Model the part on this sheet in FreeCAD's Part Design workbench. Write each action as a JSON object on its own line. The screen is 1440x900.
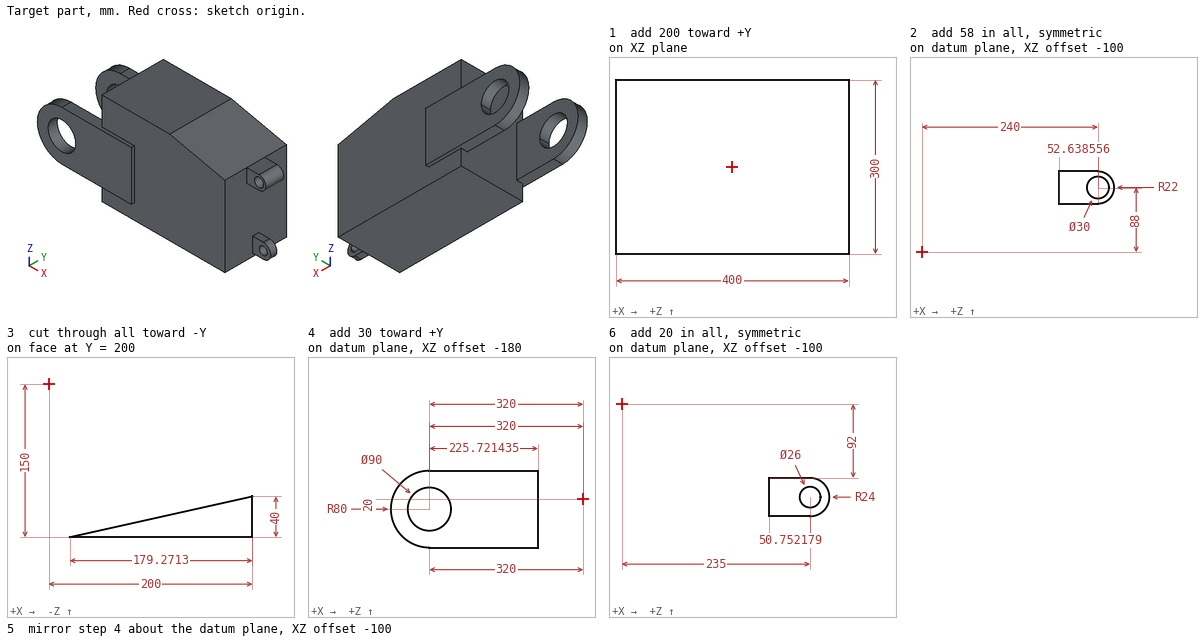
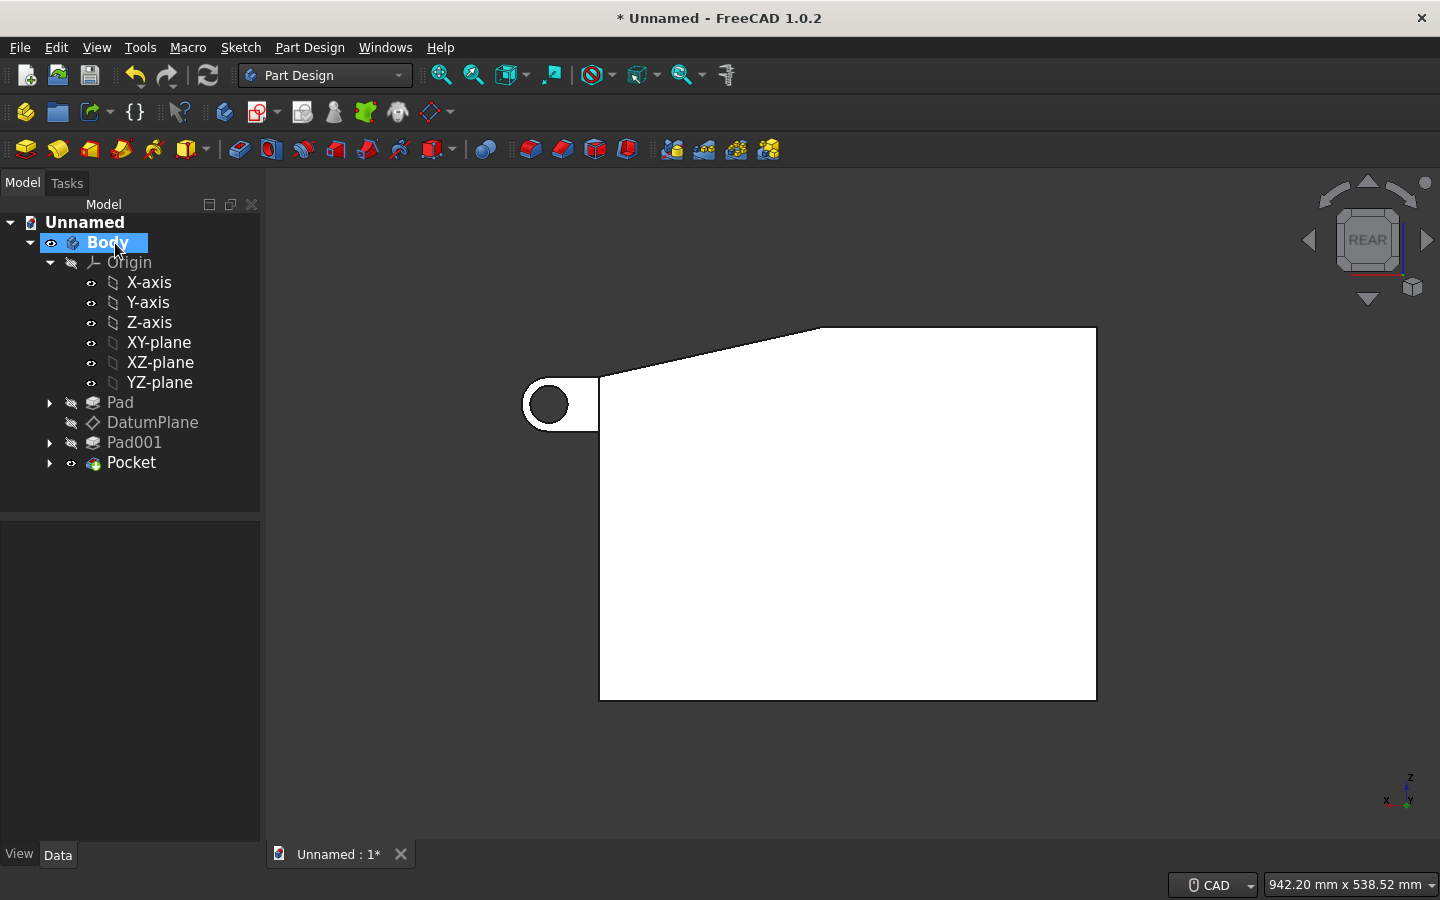
{"action": "left_click", "coordinate": [136, 363]}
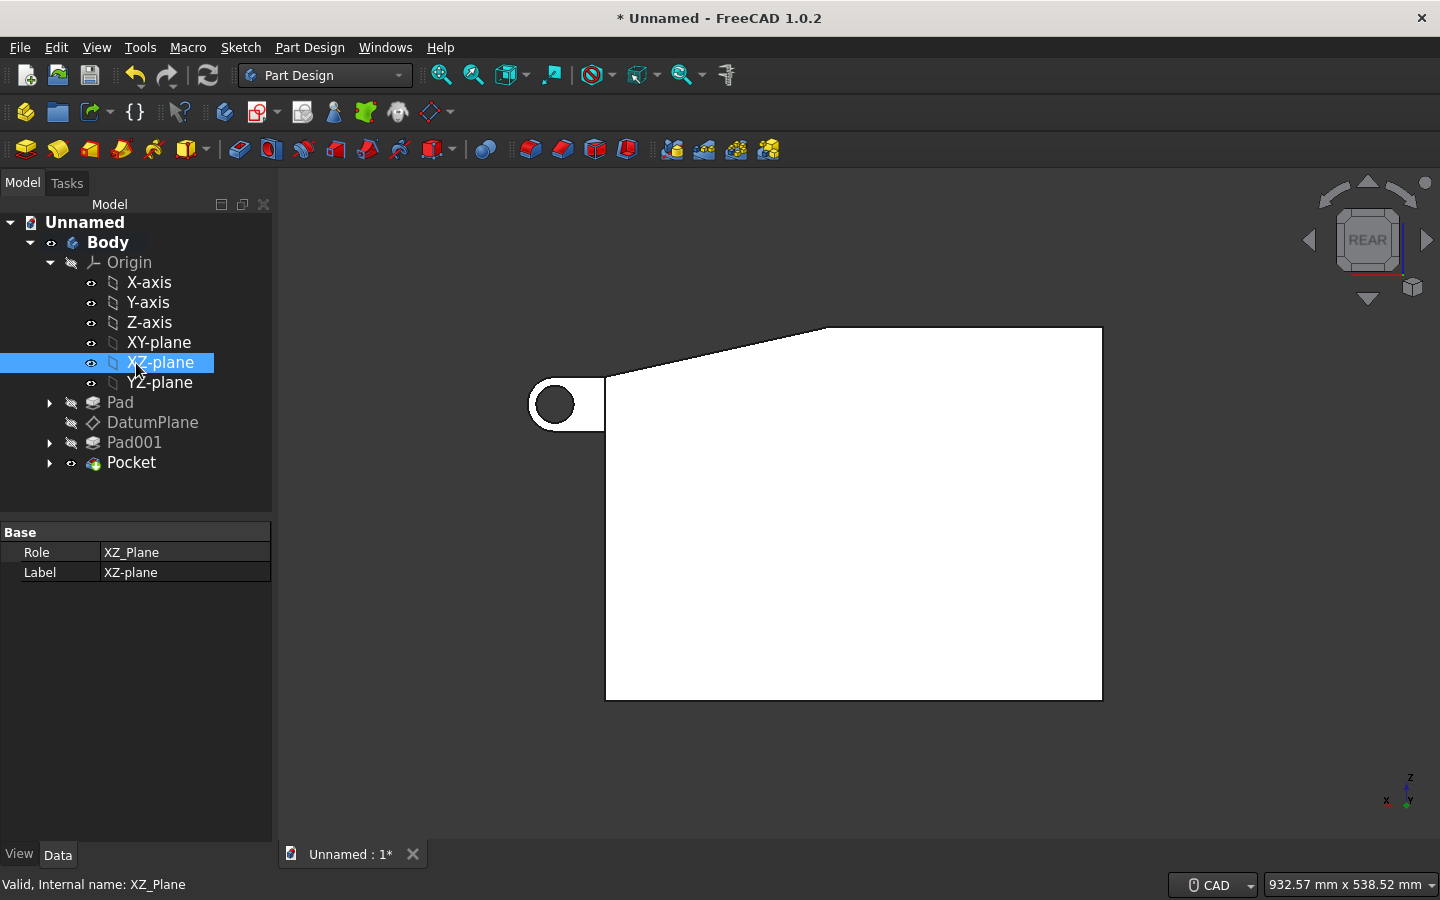
{"action": "left_click", "coordinate": [430, 112]}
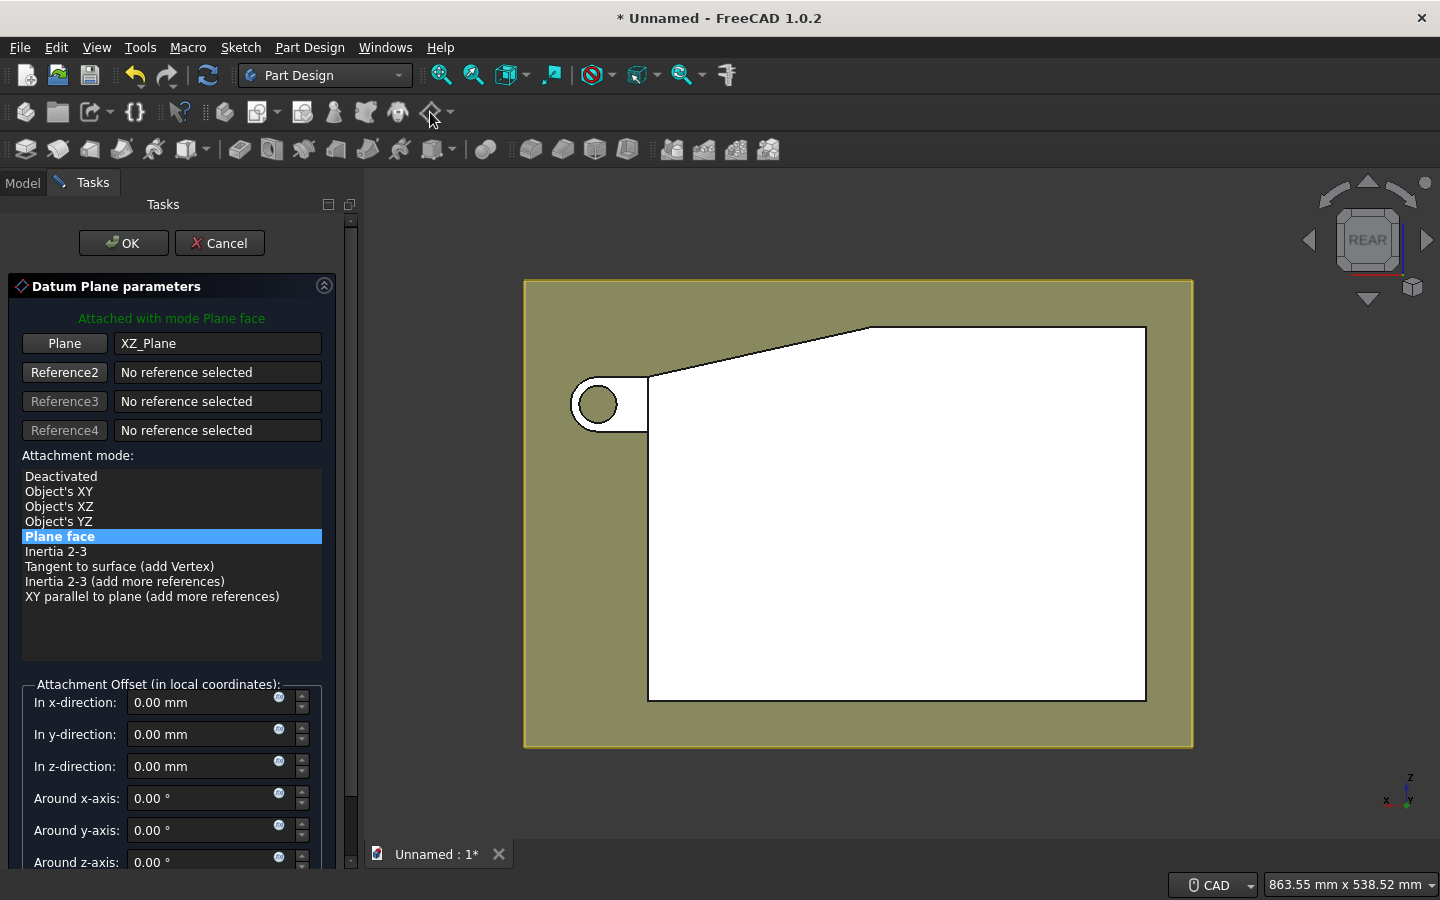
{"action": "triple_click", "coordinate": [210, 766]}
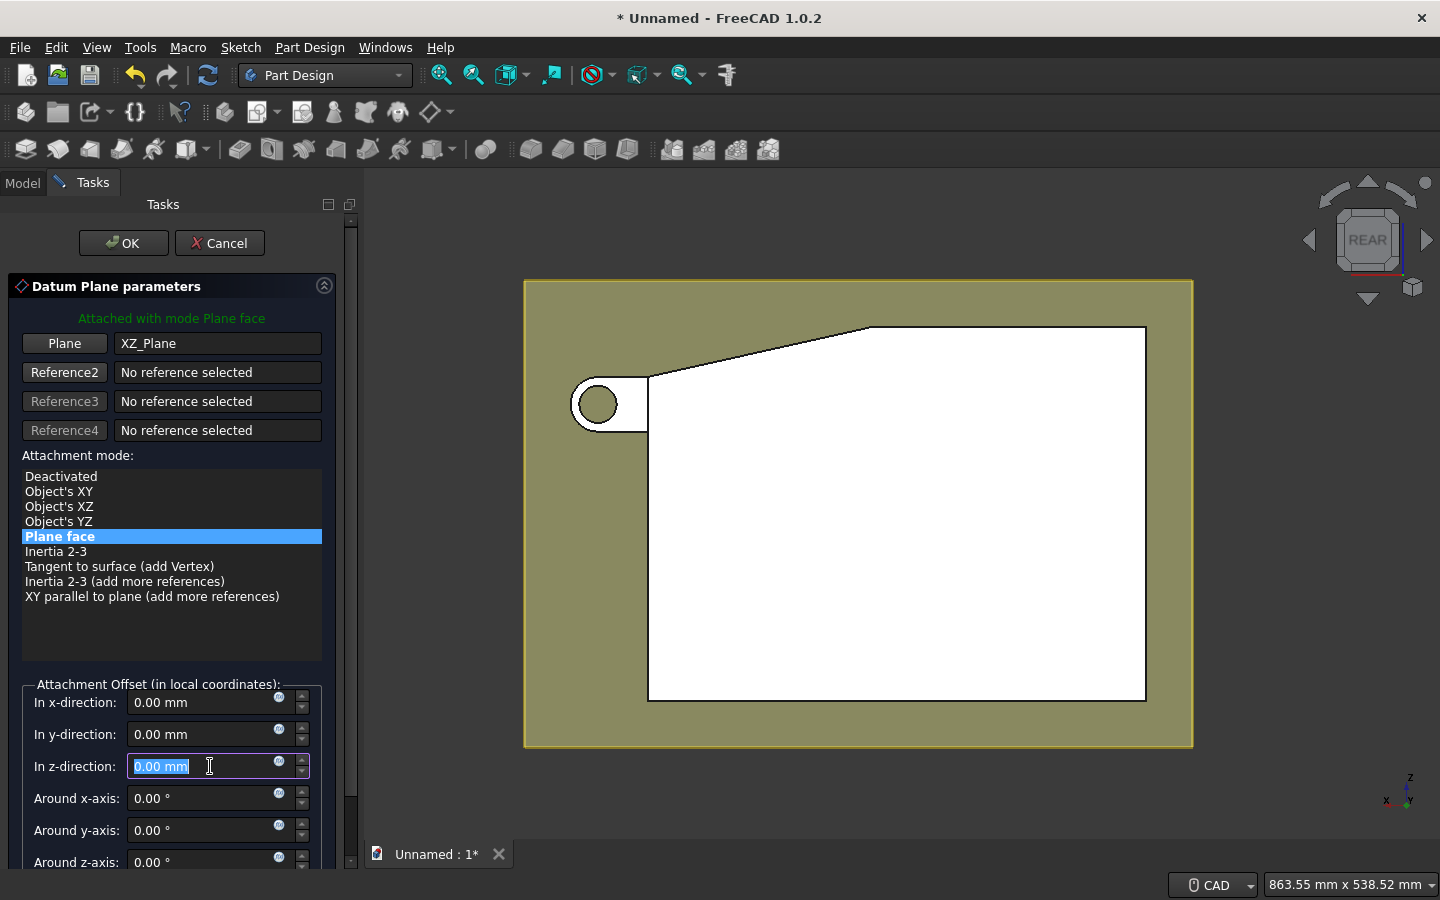
{"action": "type", "text": "-180"}
{"action": "key", "text": "Tab"}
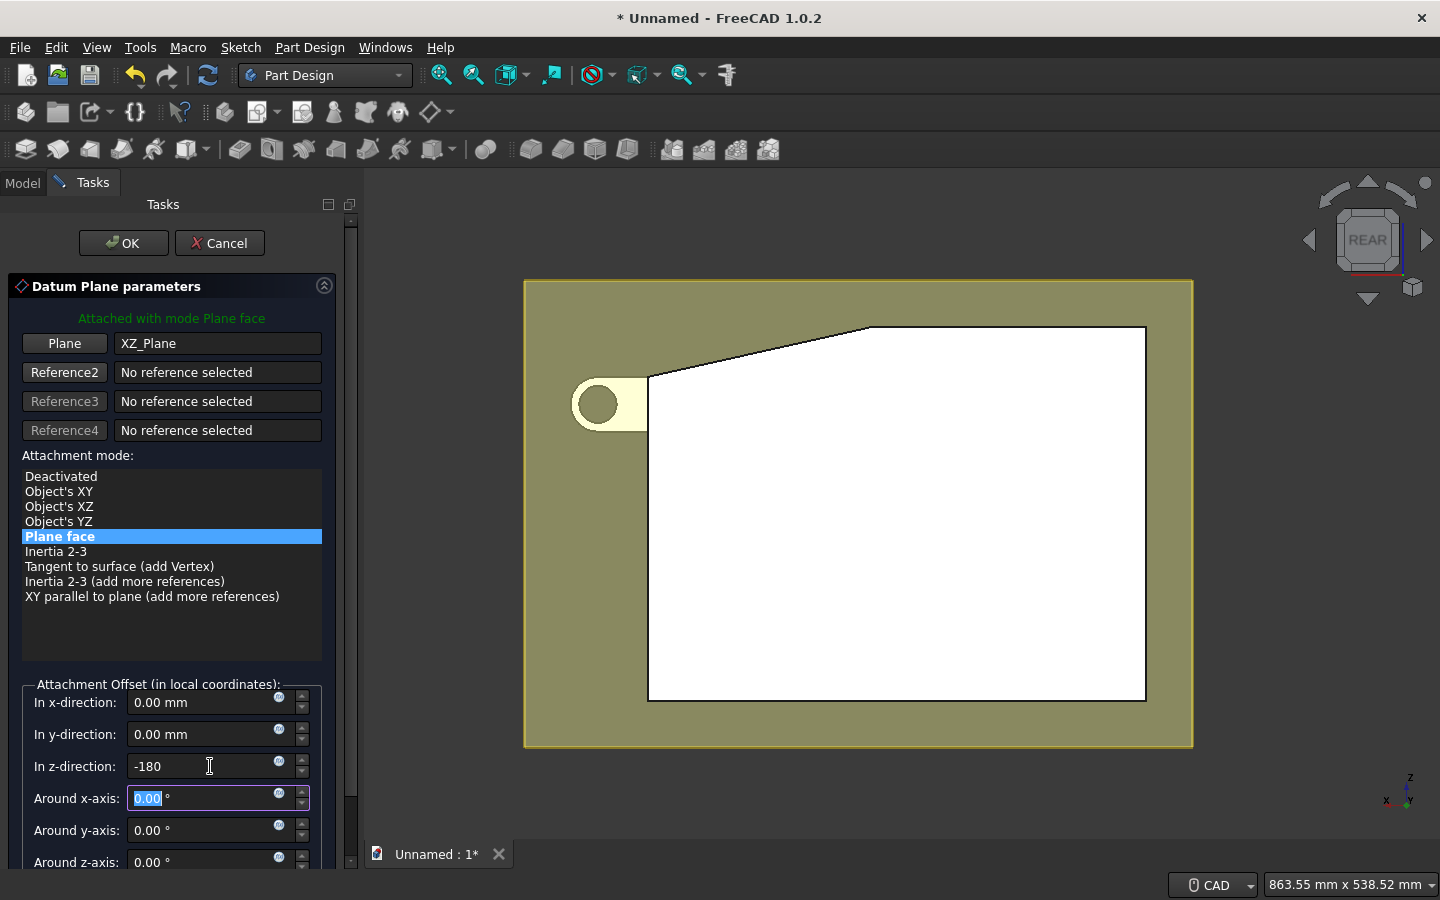
{"action": "left_click", "coordinate": [124, 243]}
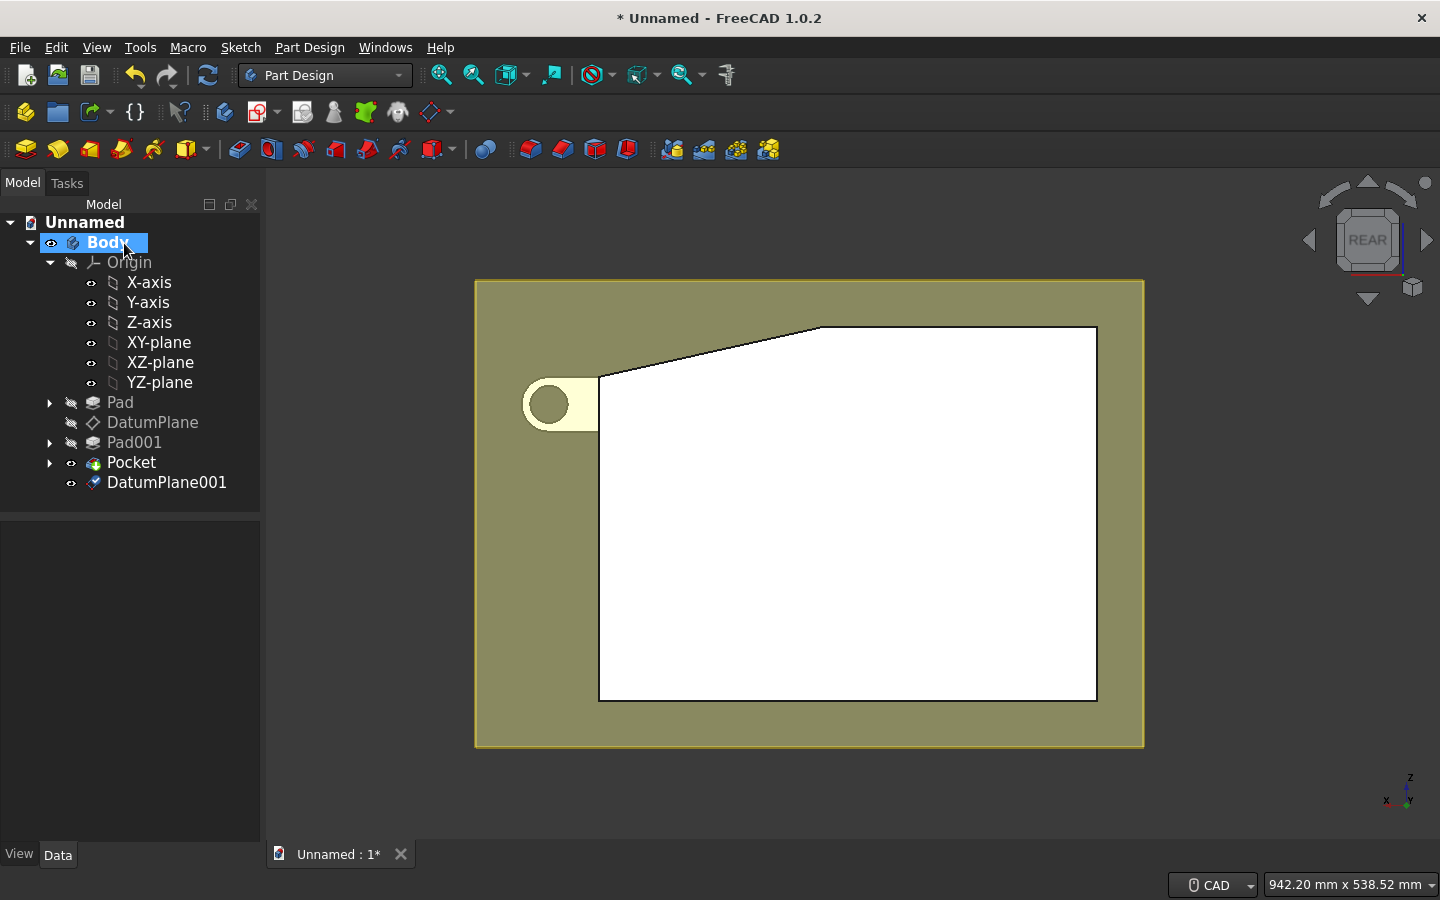
{"action": "left_click", "coordinate": [116, 483]}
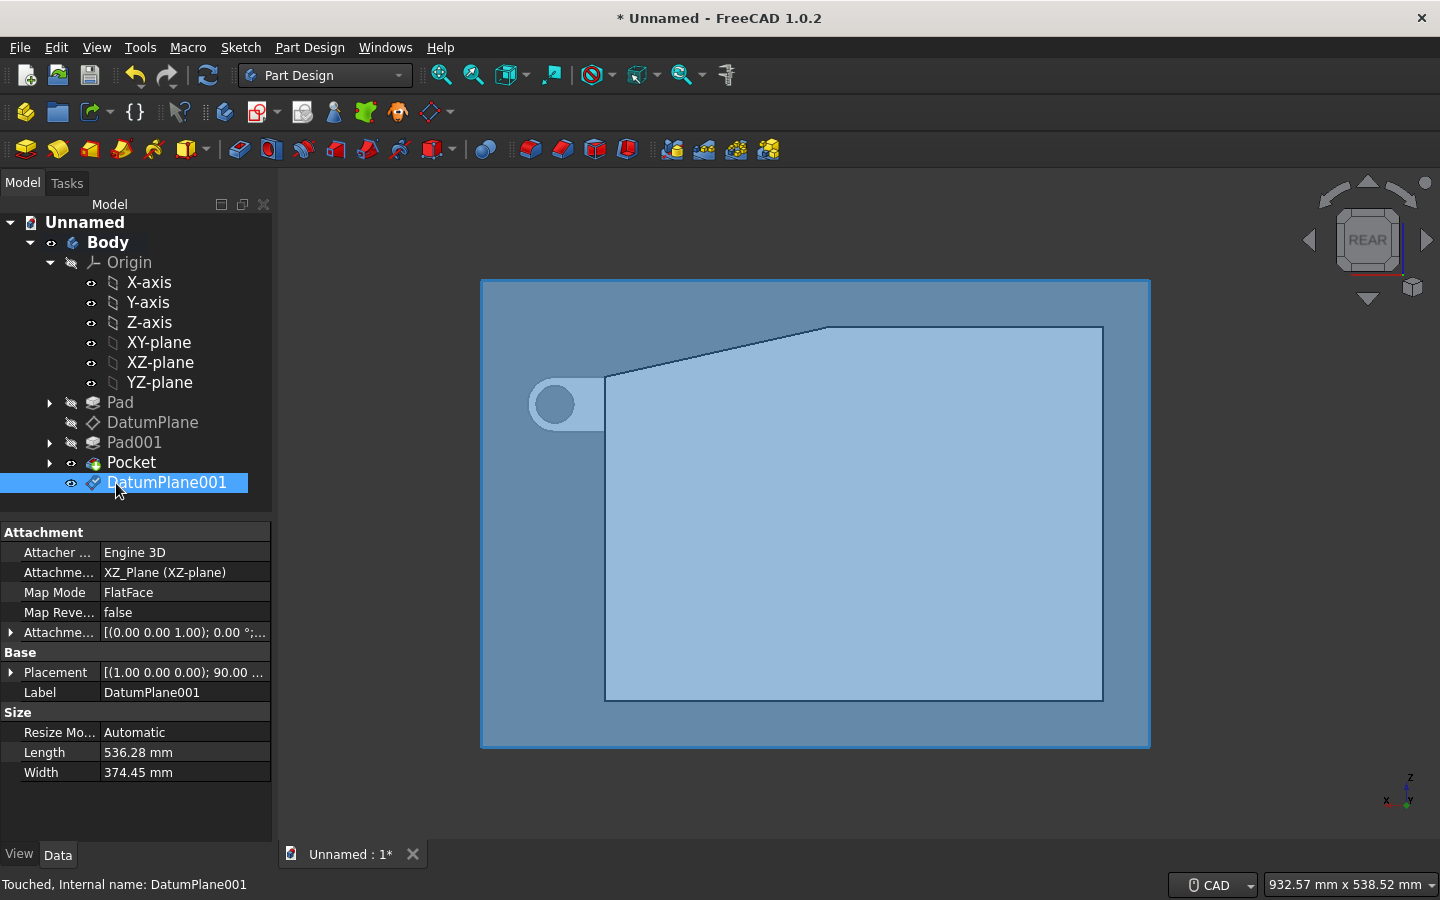
{"action": "left_click", "coordinate": [258, 112]}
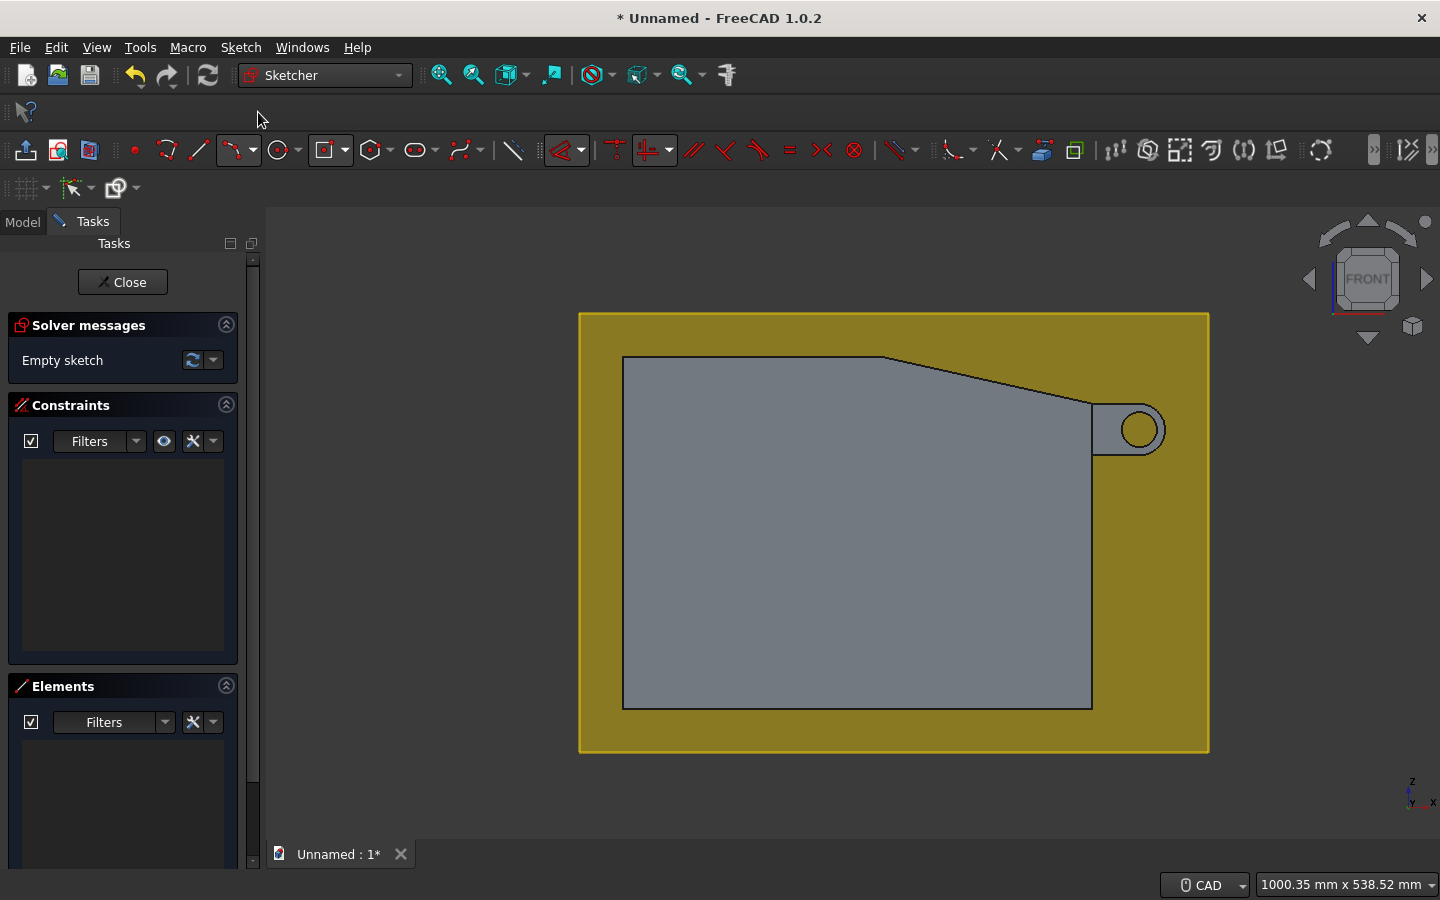
{"action": "left_click", "coordinate": [90, 150]}